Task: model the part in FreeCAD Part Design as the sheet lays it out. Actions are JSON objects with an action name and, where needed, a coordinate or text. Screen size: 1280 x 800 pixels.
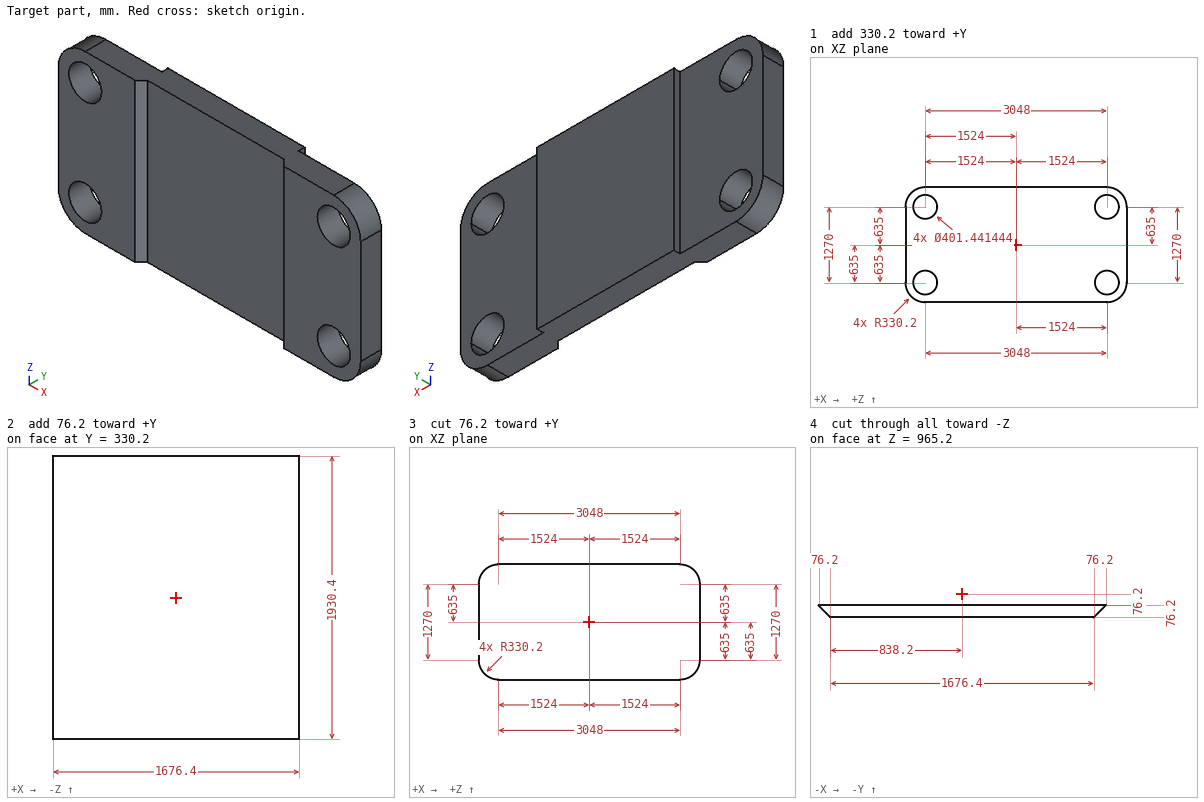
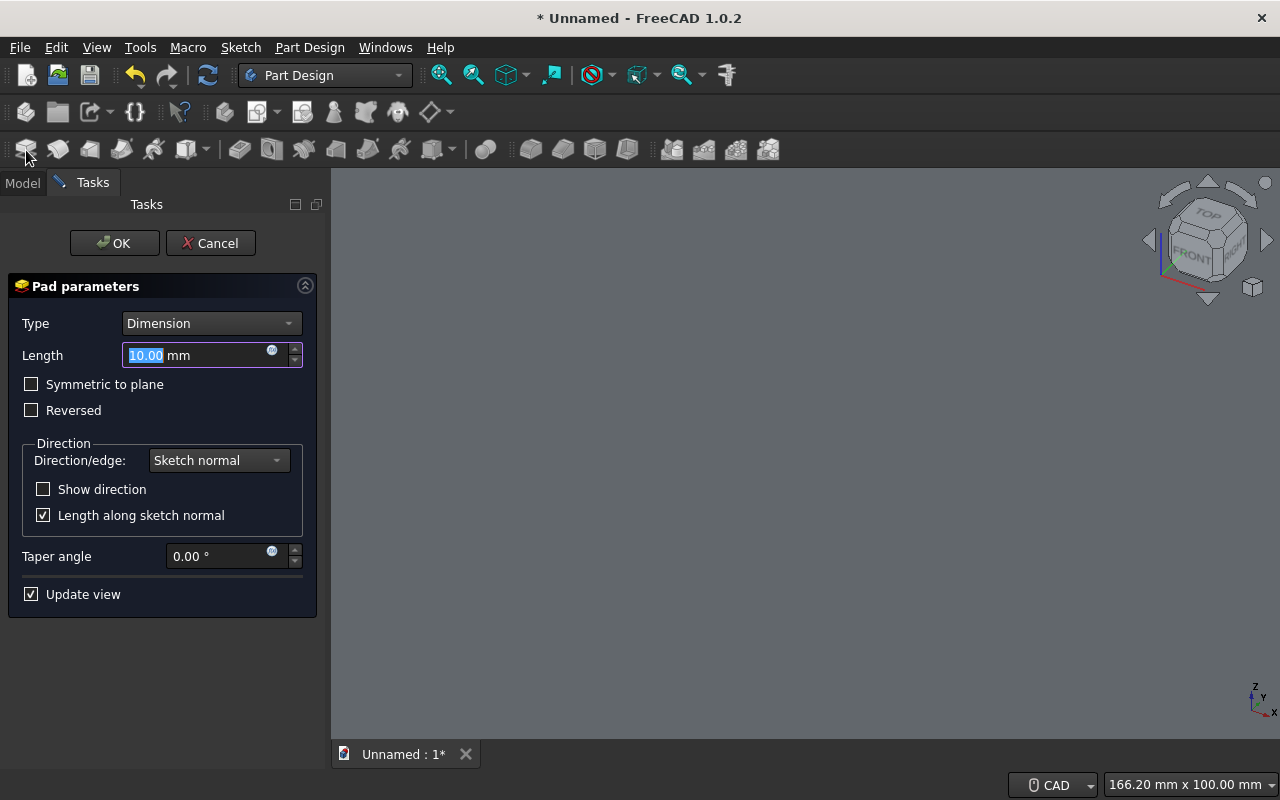
{"action": "type", "text": "330.2"}
{"action": "key", "text": "Tab"}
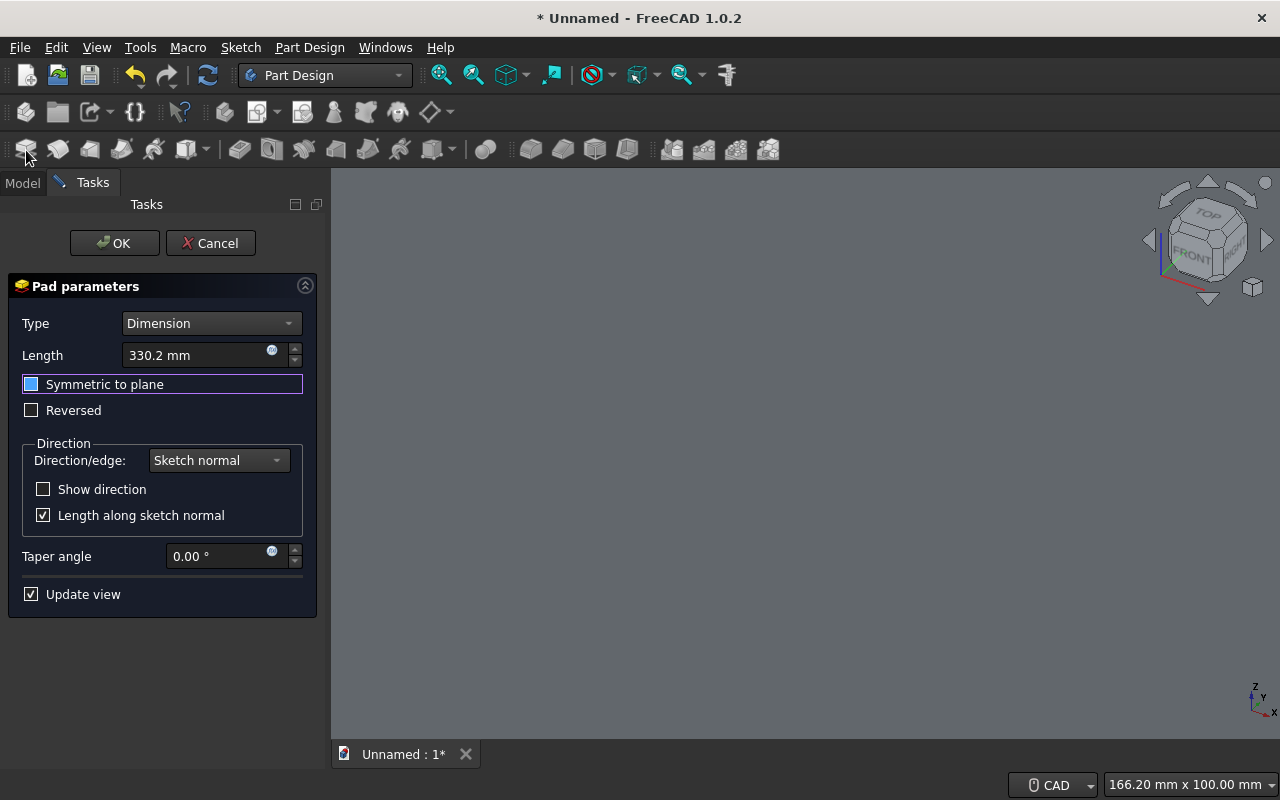
{"action": "left_click", "coordinate": [30, 410]}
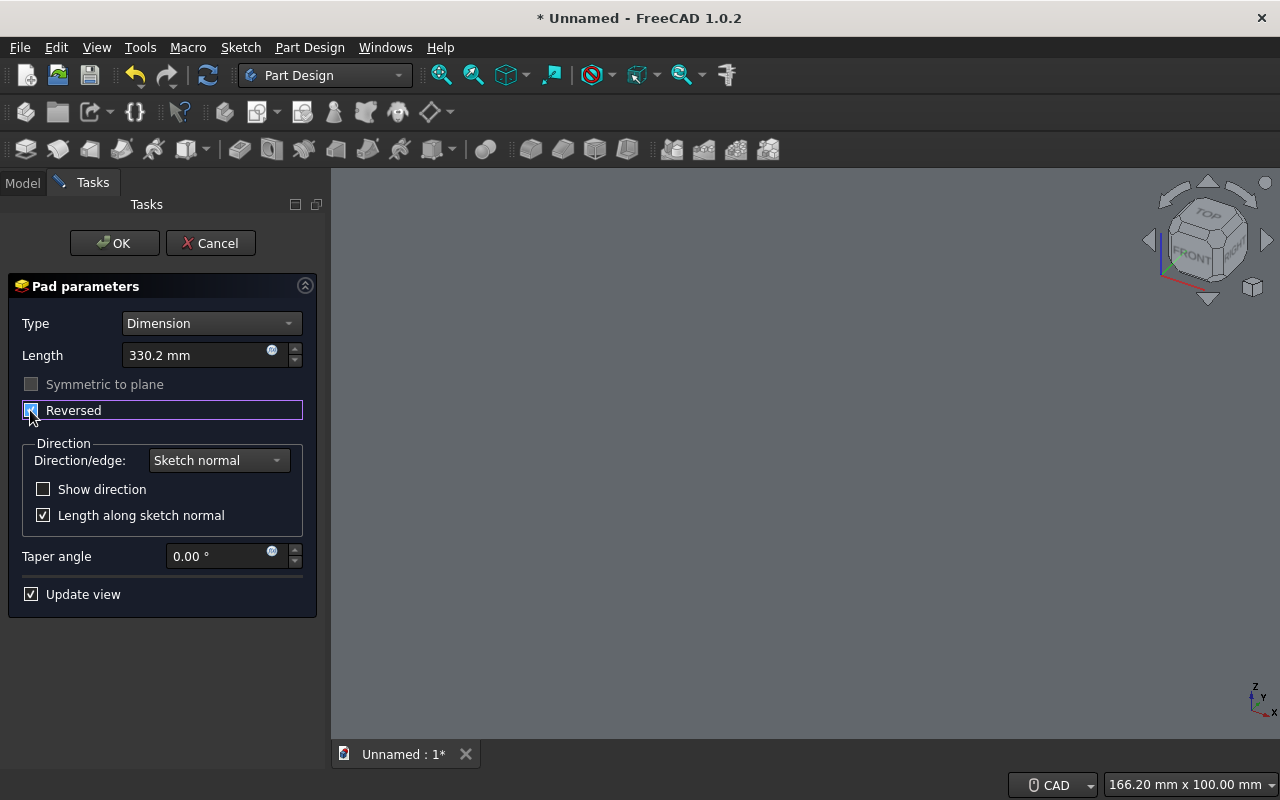
{"action": "left_click", "coordinate": [115, 243]}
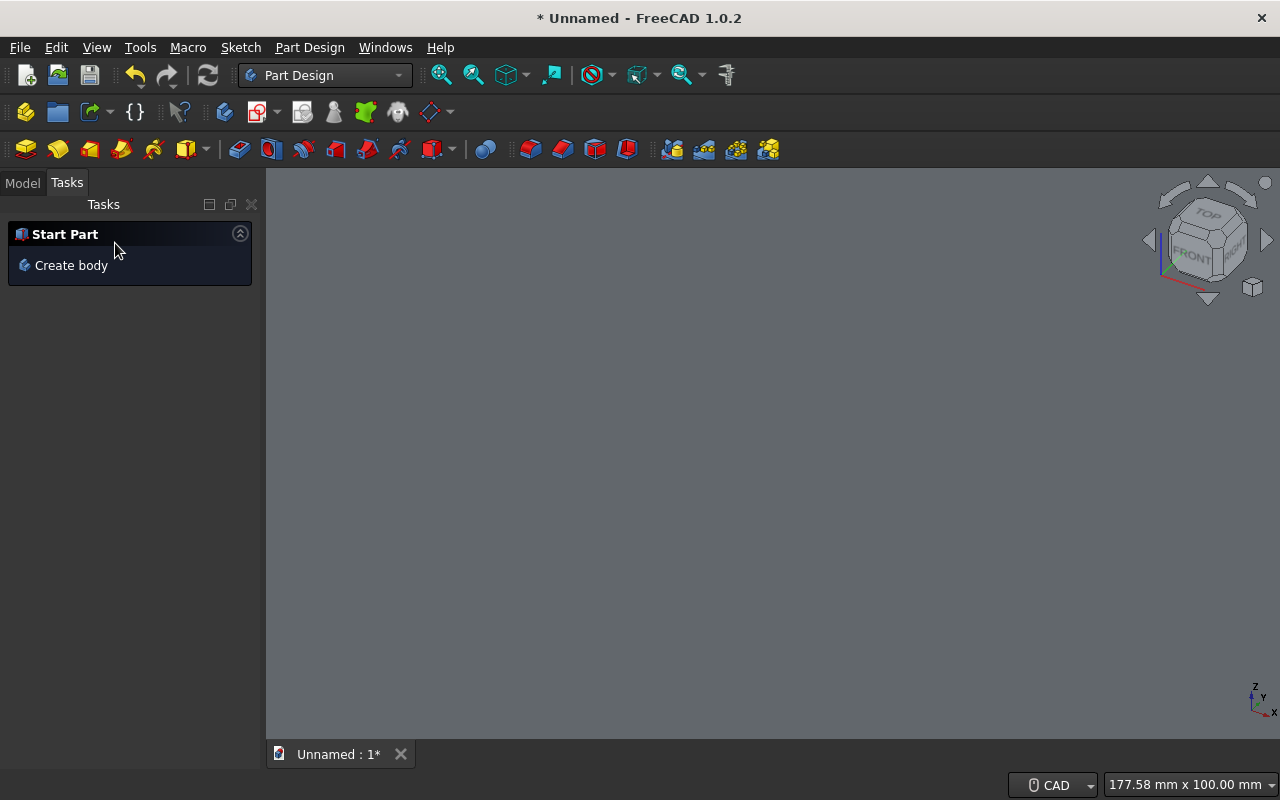
{"action": "key", "text": "v f"}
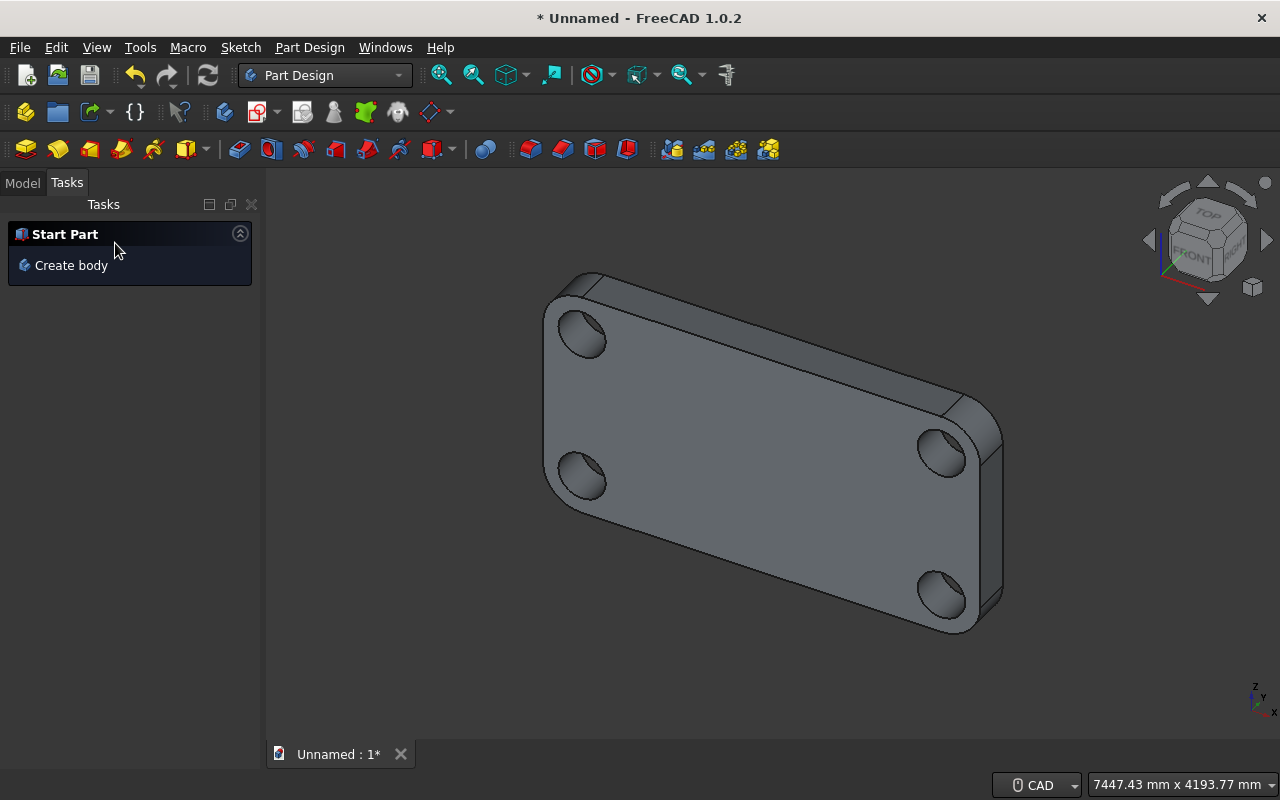
{"action": "key", "text": "4"}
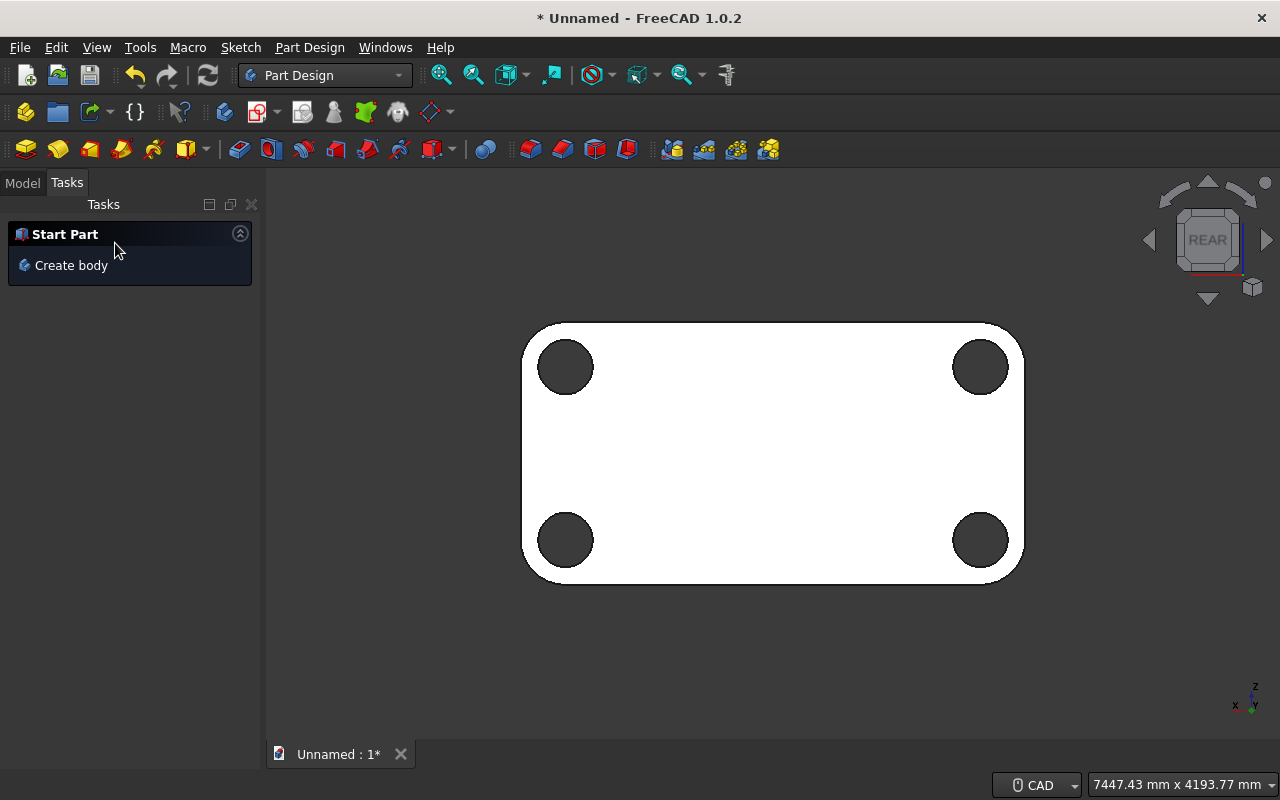
{"action": "left_click", "coordinate": [701, 452]}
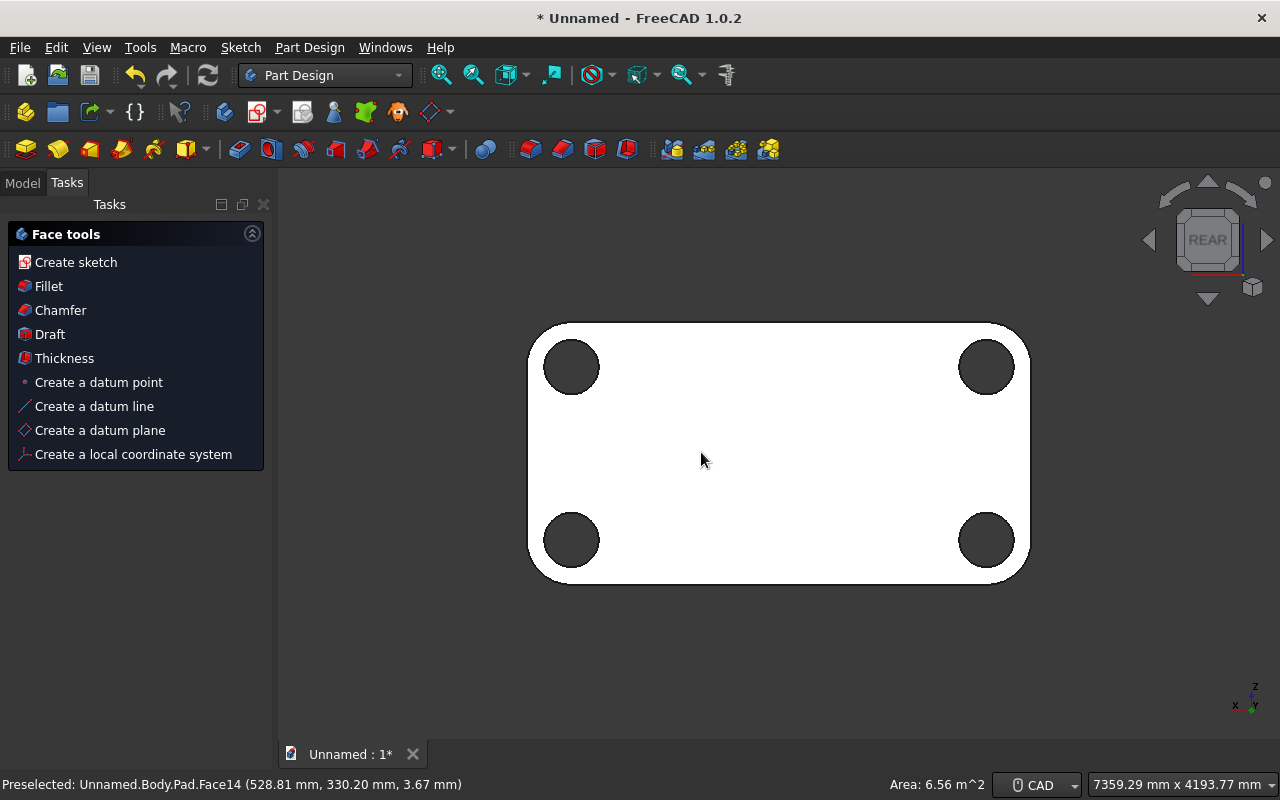
{"action": "left_click", "coordinate": [258, 112]}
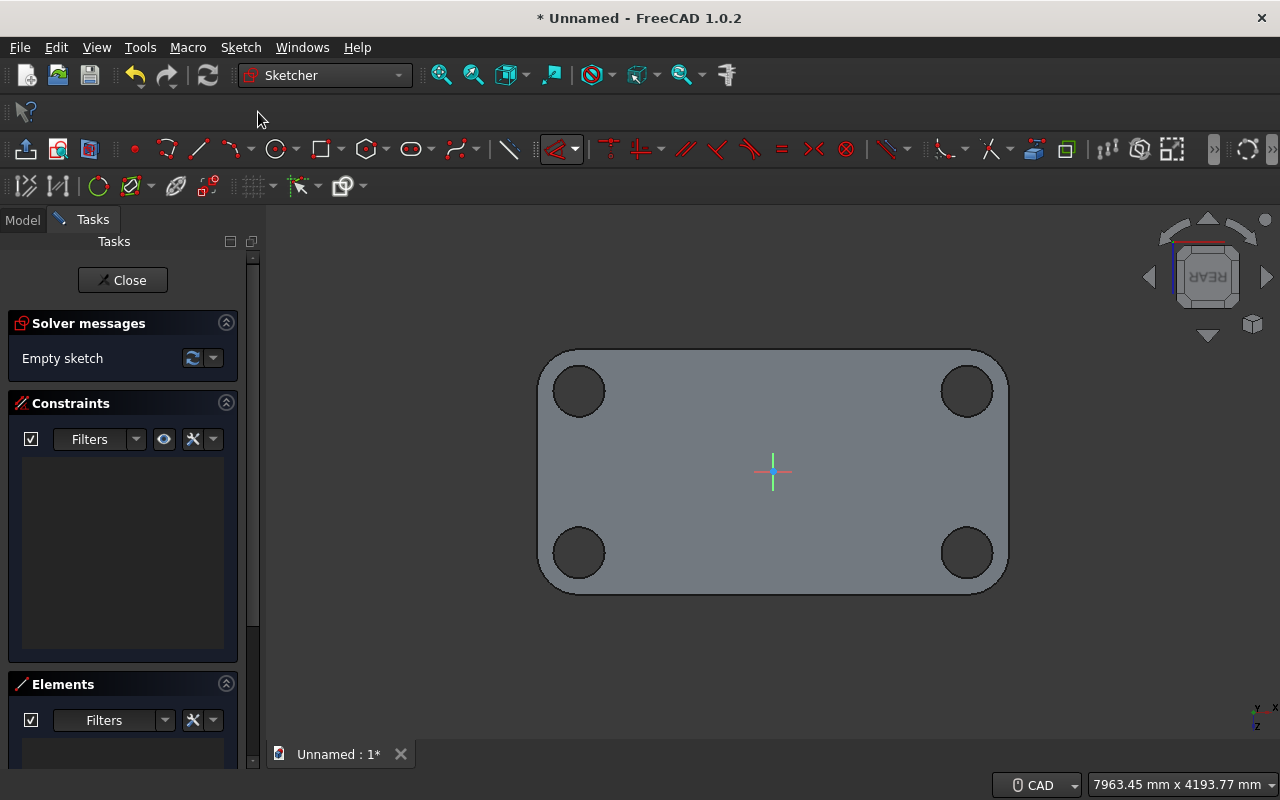
{"action": "scroll", "coordinate": [912, 472], "scroll_direction": "up", "scroll_amount": 2}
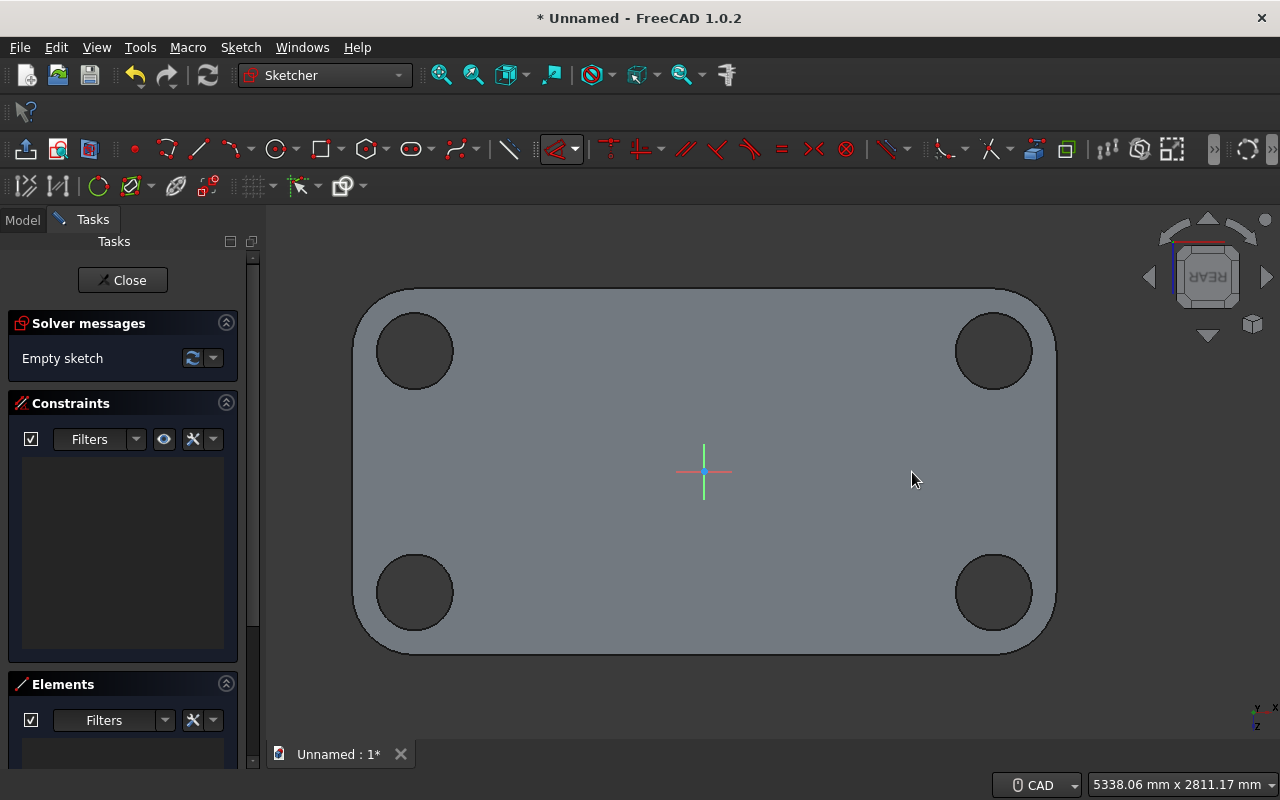
{"action": "key", "text": "g v"}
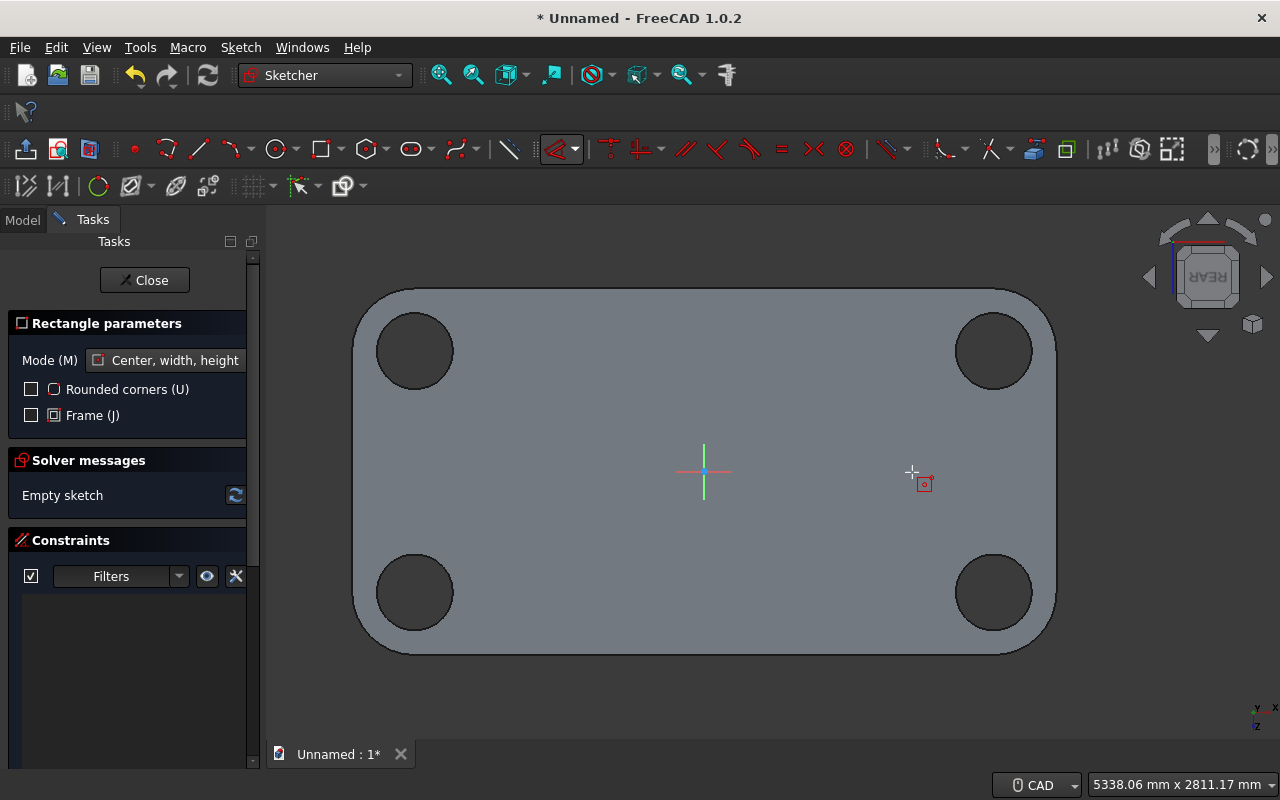
{"action": "left_click", "coordinate": [704, 472]}
{"action": "left_click", "coordinate": [864, 288]}
{"action": "key", "text": "Escape"}